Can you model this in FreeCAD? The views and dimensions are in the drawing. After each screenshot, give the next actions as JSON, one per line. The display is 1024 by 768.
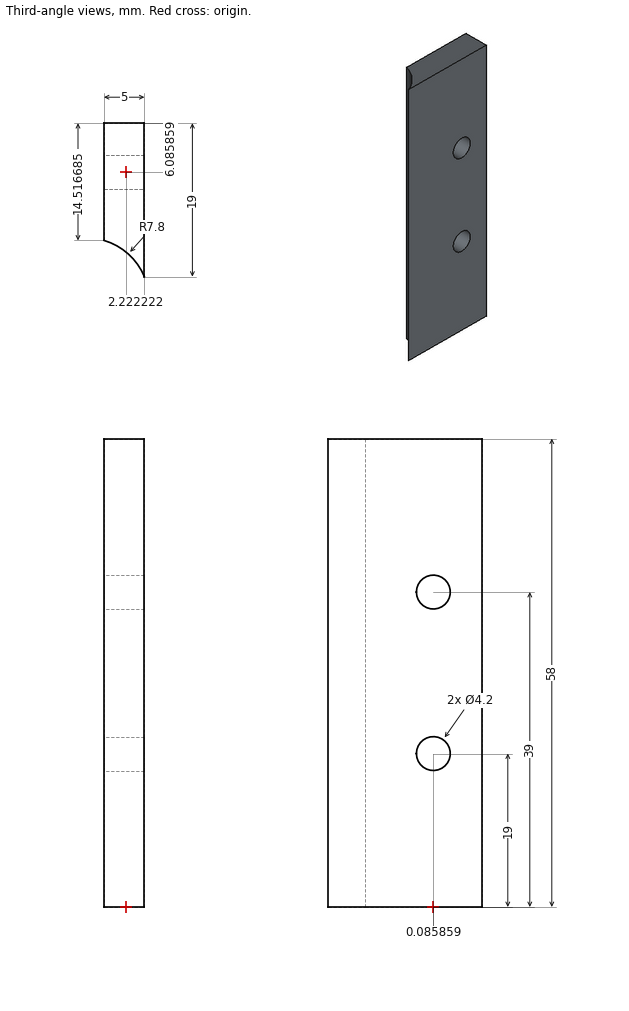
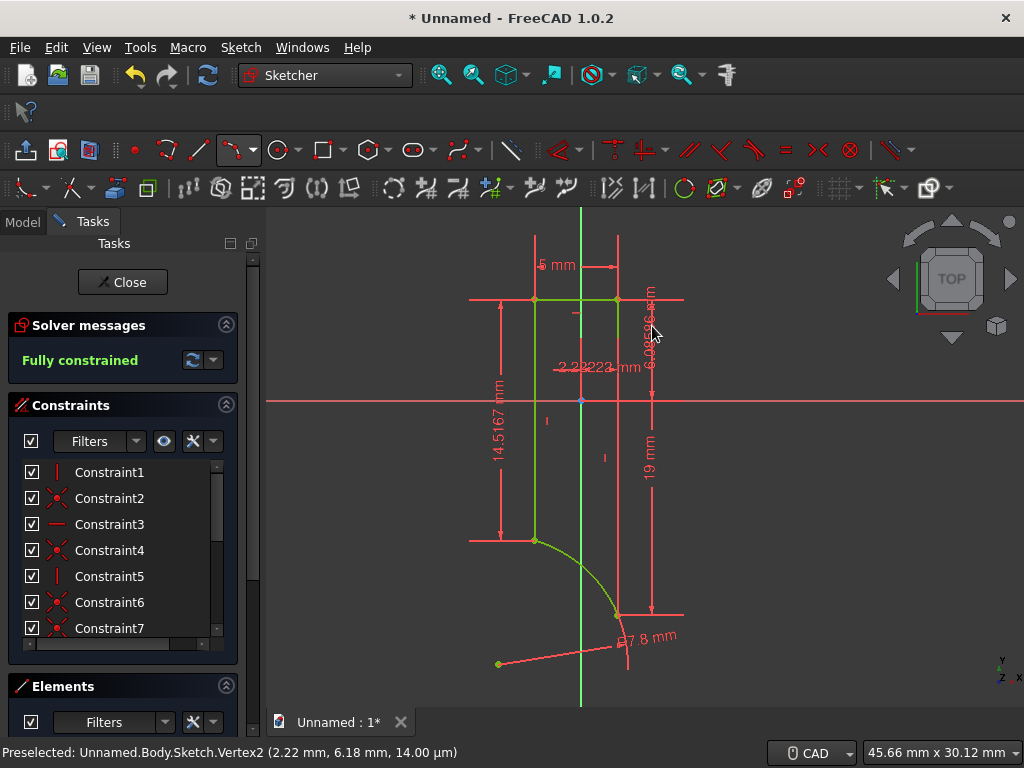
{"action": "left_click", "coordinate": [123, 282]}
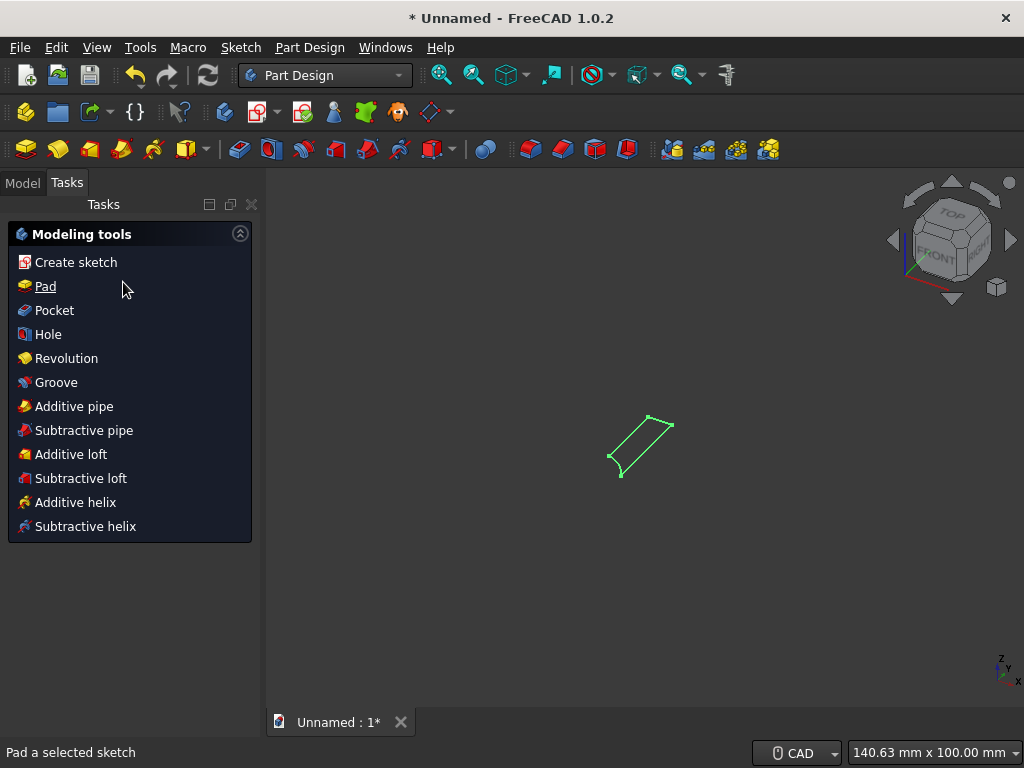
{"action": "left_click", "coordinate": [26, 150]}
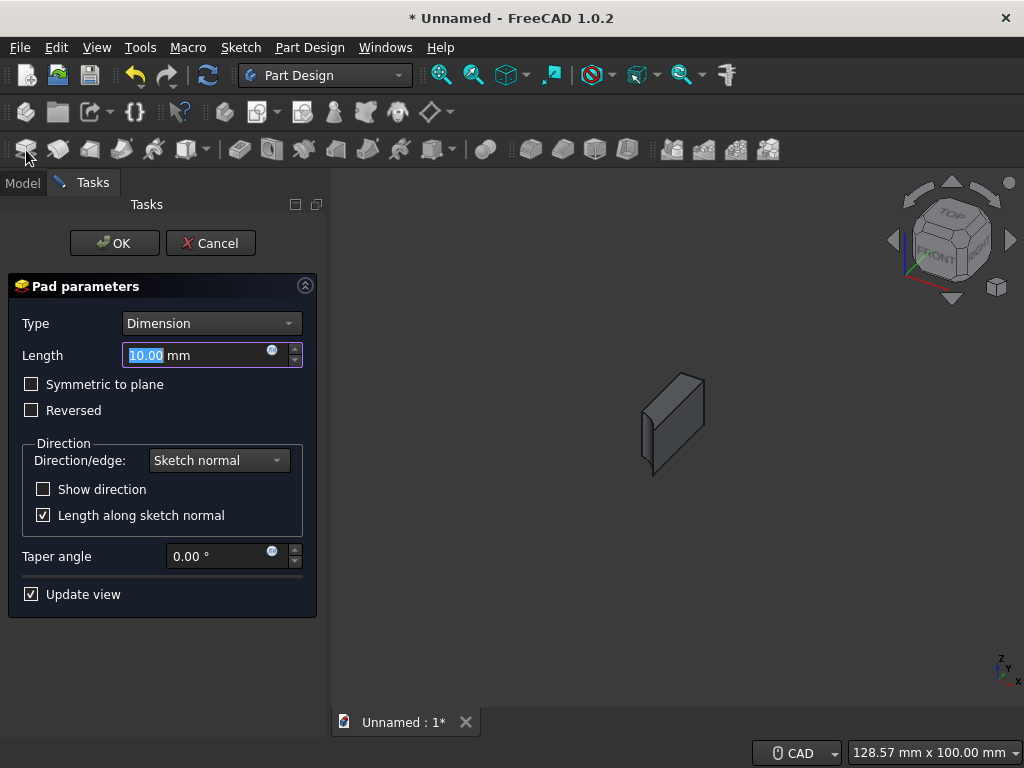
{"action": "type", "text": "58"}
{"action": "key", "text": "Tab"}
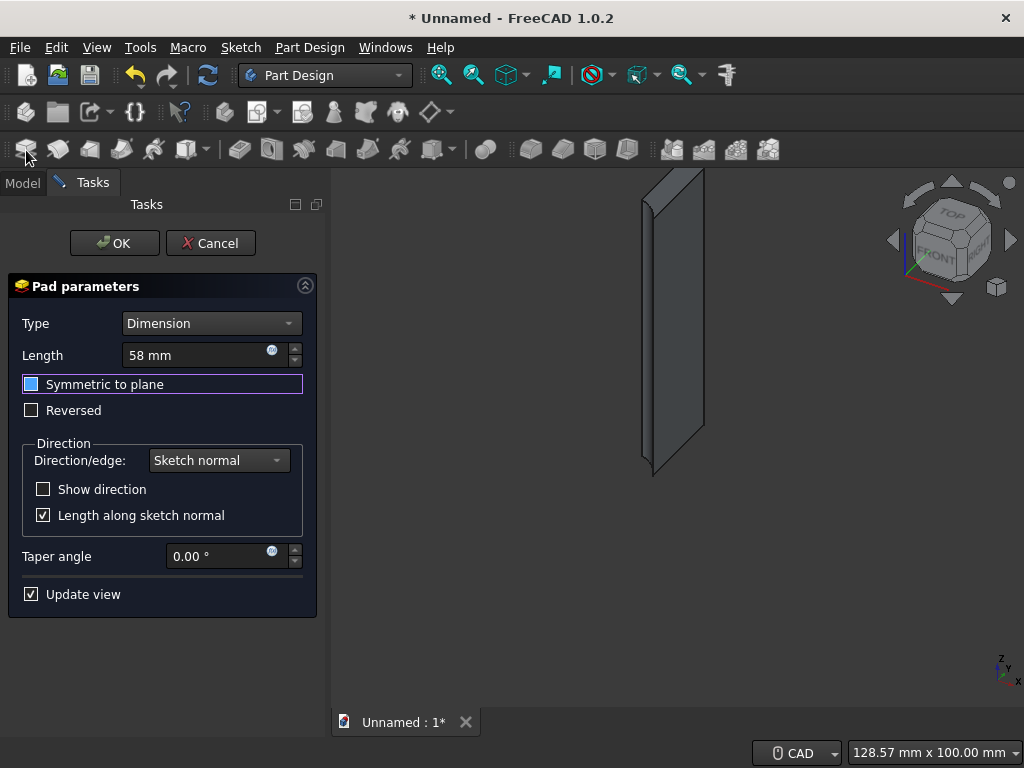
{"action": "left_click", "coordinate": [115, 243]}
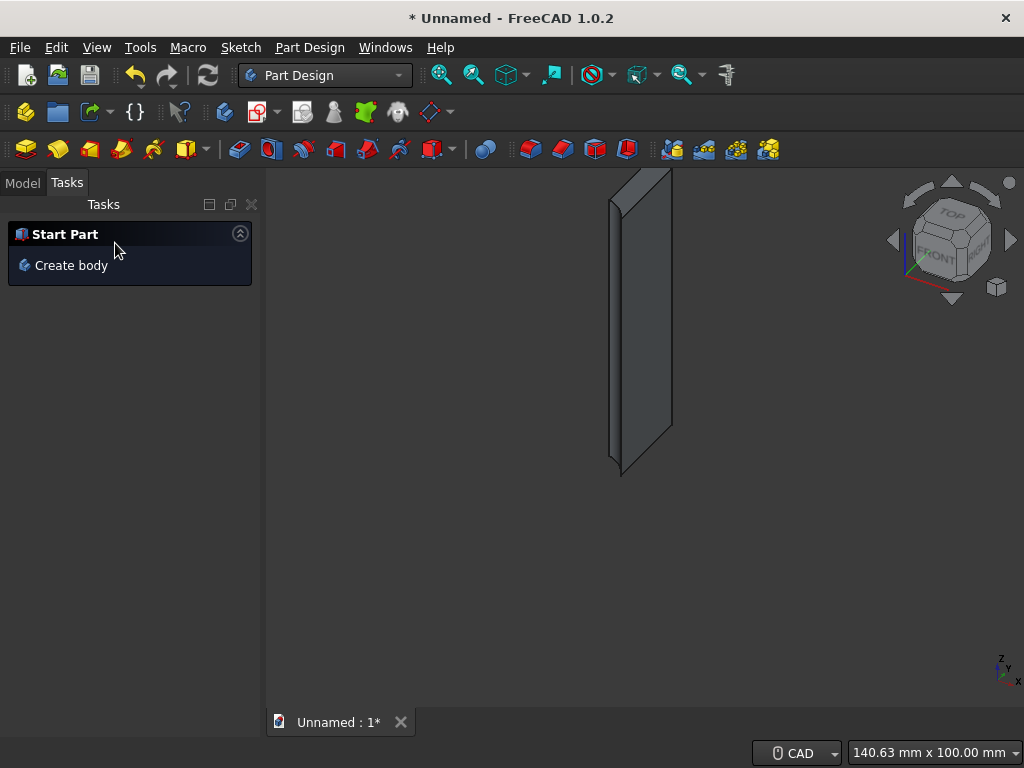
{"action": "left_click", "coordinate": [442, 76]}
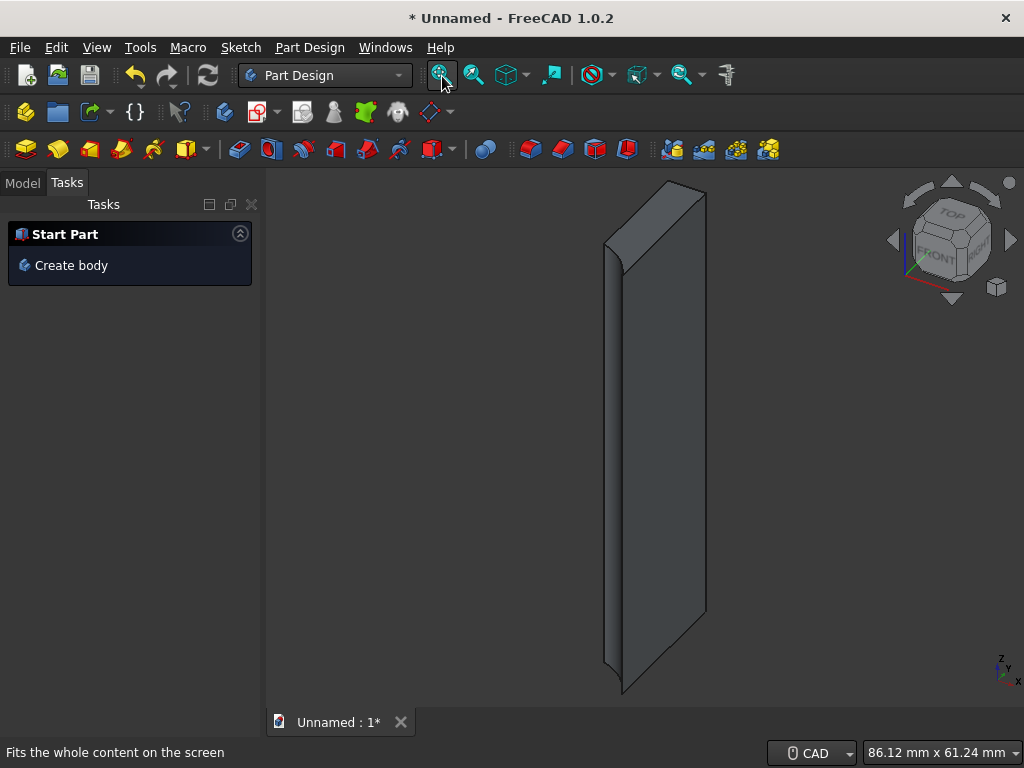
{"action": "key", "text": "6"}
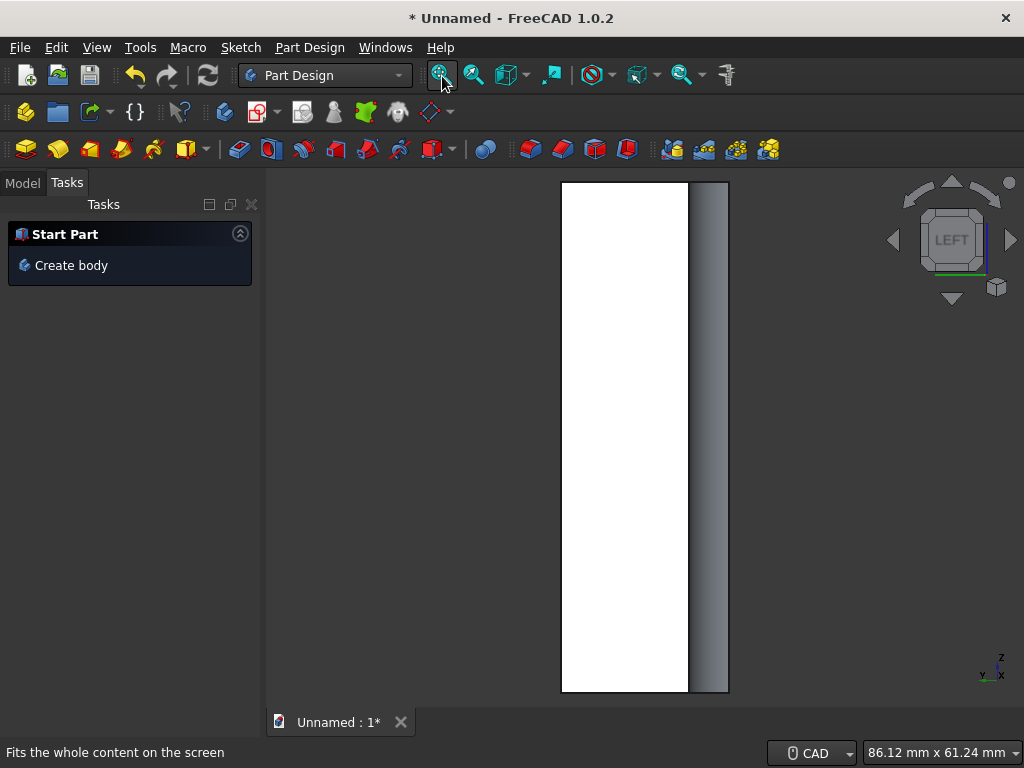
{"action": "left_click", "coordinate": [625, 291]}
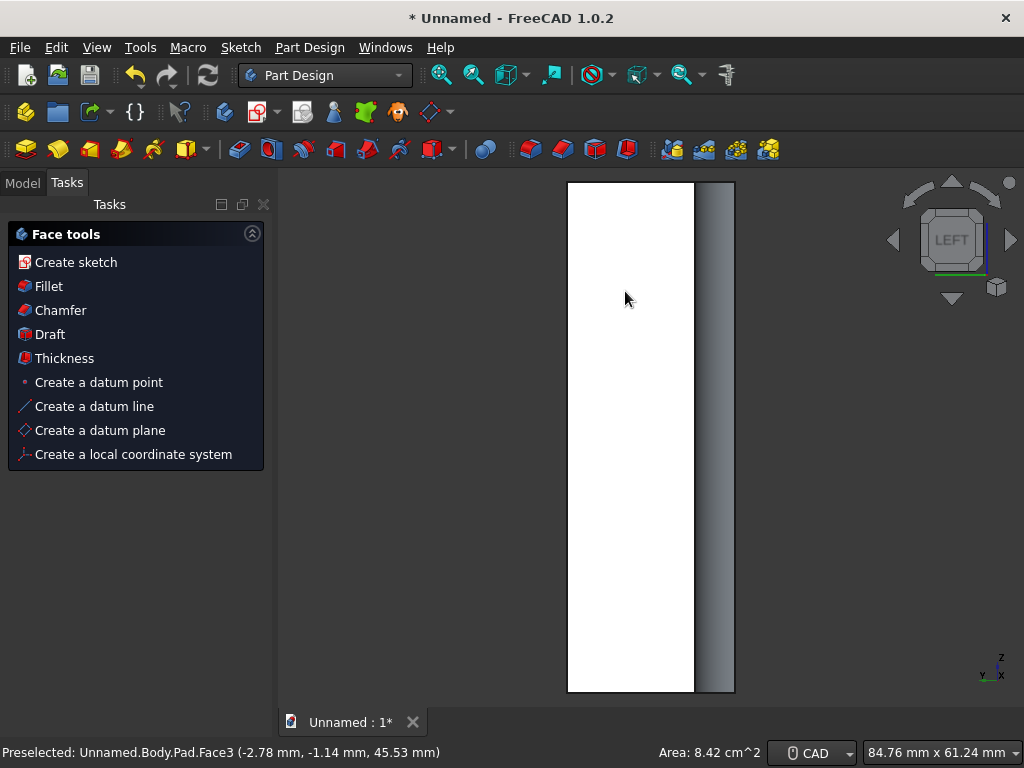
{"action": "left_click", "coordinate": [258, 112]}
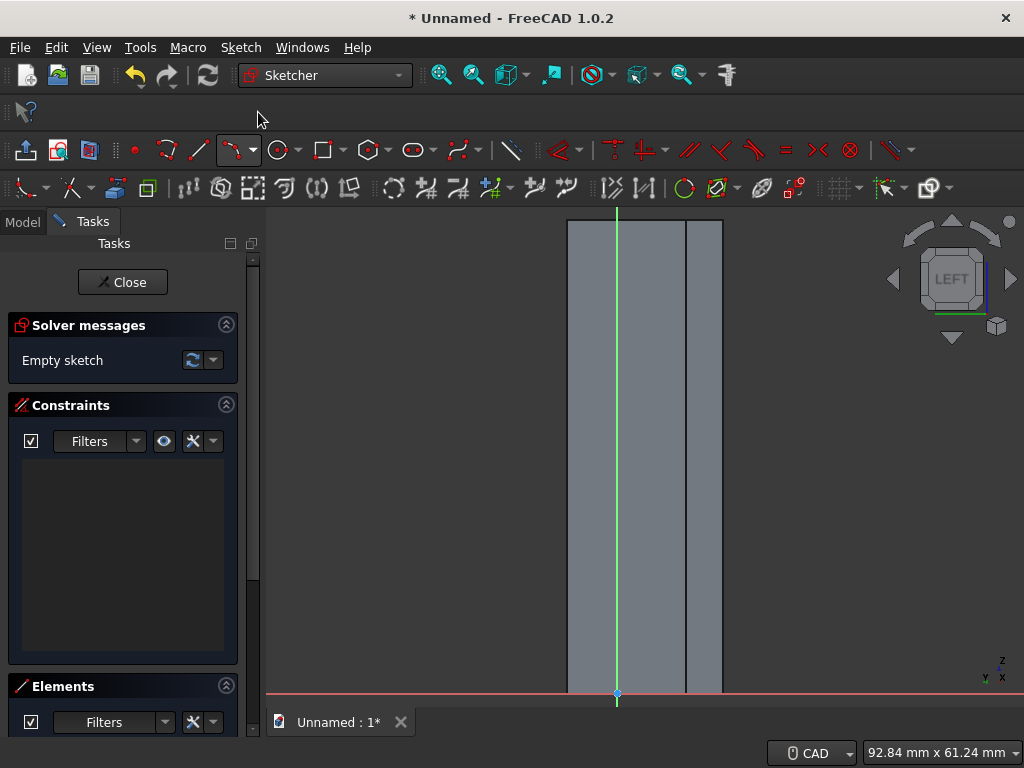
{"action": "scroll", "coordinate": [396, 235], "scroll_direction": "down", "scroll_amount": 1}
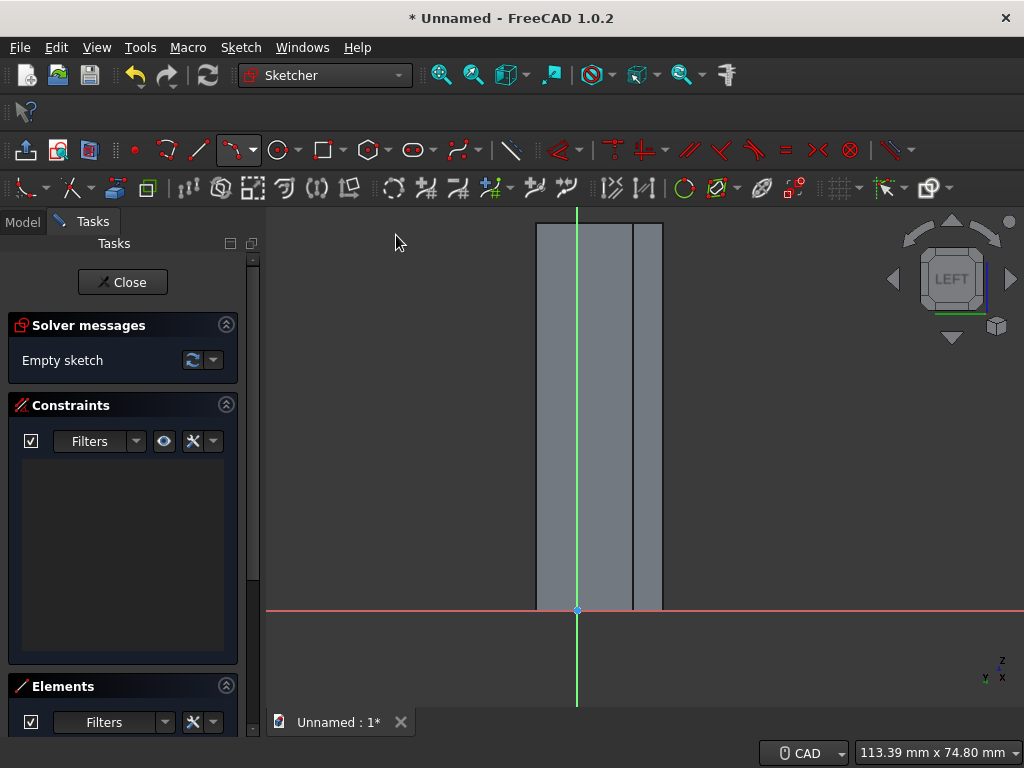
{"action": "left_click", "coordinate": [278, 150]}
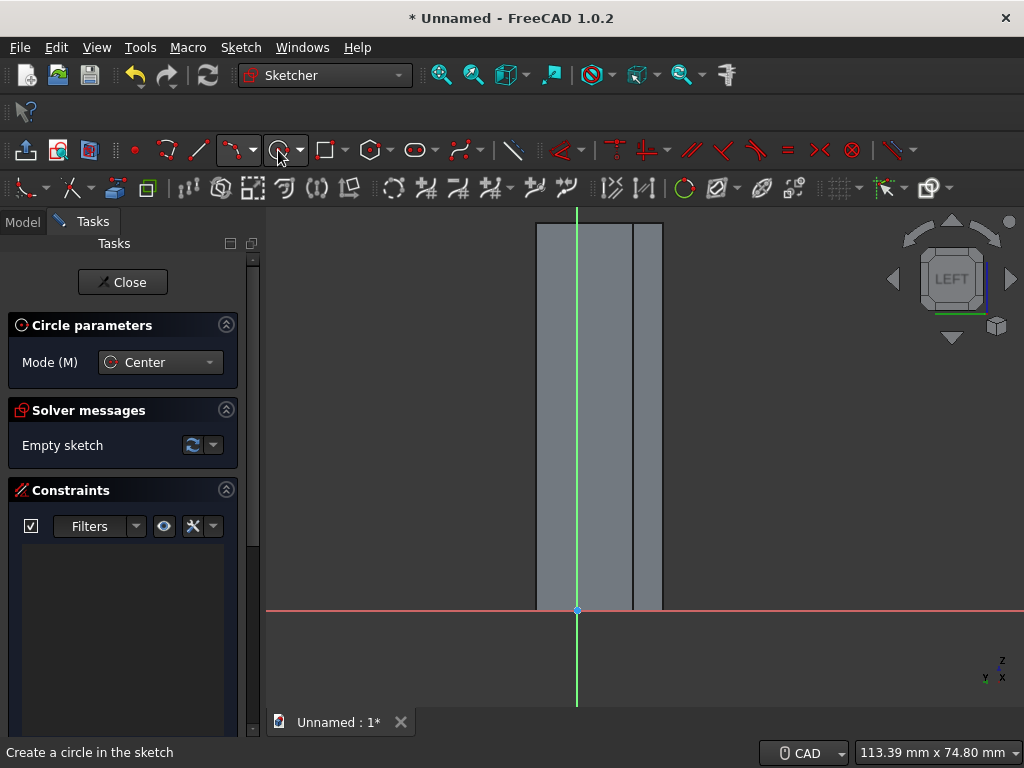
{"action": "scroll", "coordinate": [576, 484], "scroll_direction": "up", "scroll_amount": 17}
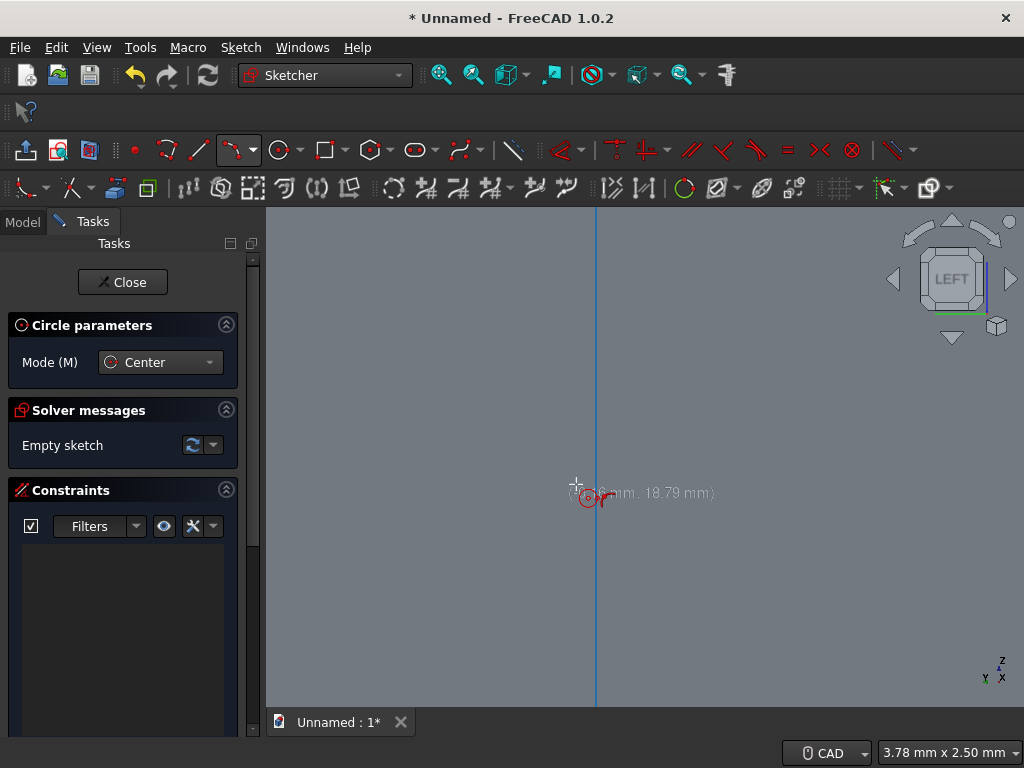
{"action": "left_click", "coordinate": [579, 456]}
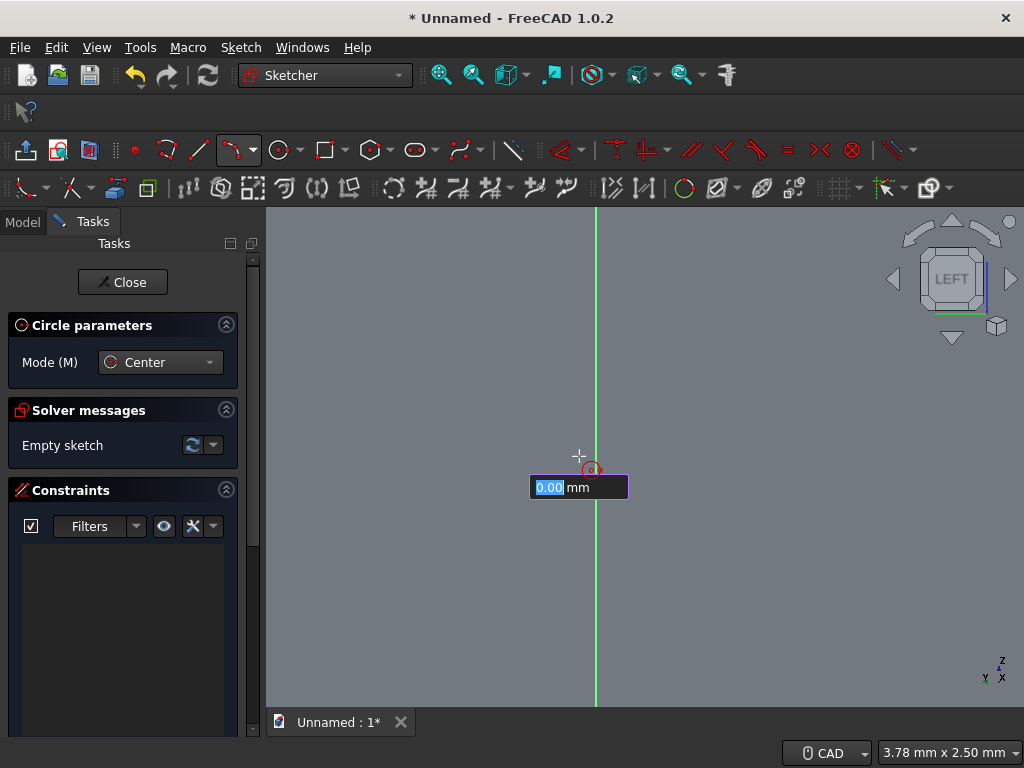
{"action": "scroll", "coordinate": [576, 470], "scroll_direction": "down", "scroll_amount": 16}